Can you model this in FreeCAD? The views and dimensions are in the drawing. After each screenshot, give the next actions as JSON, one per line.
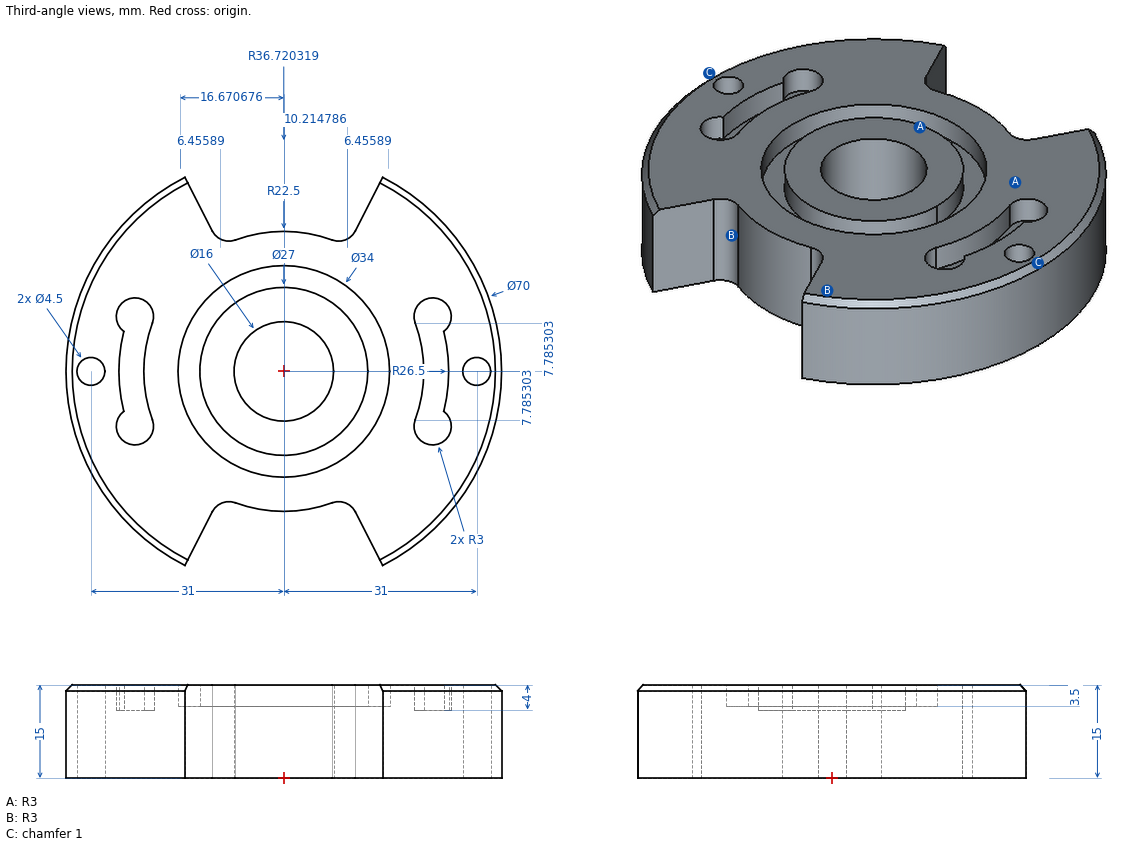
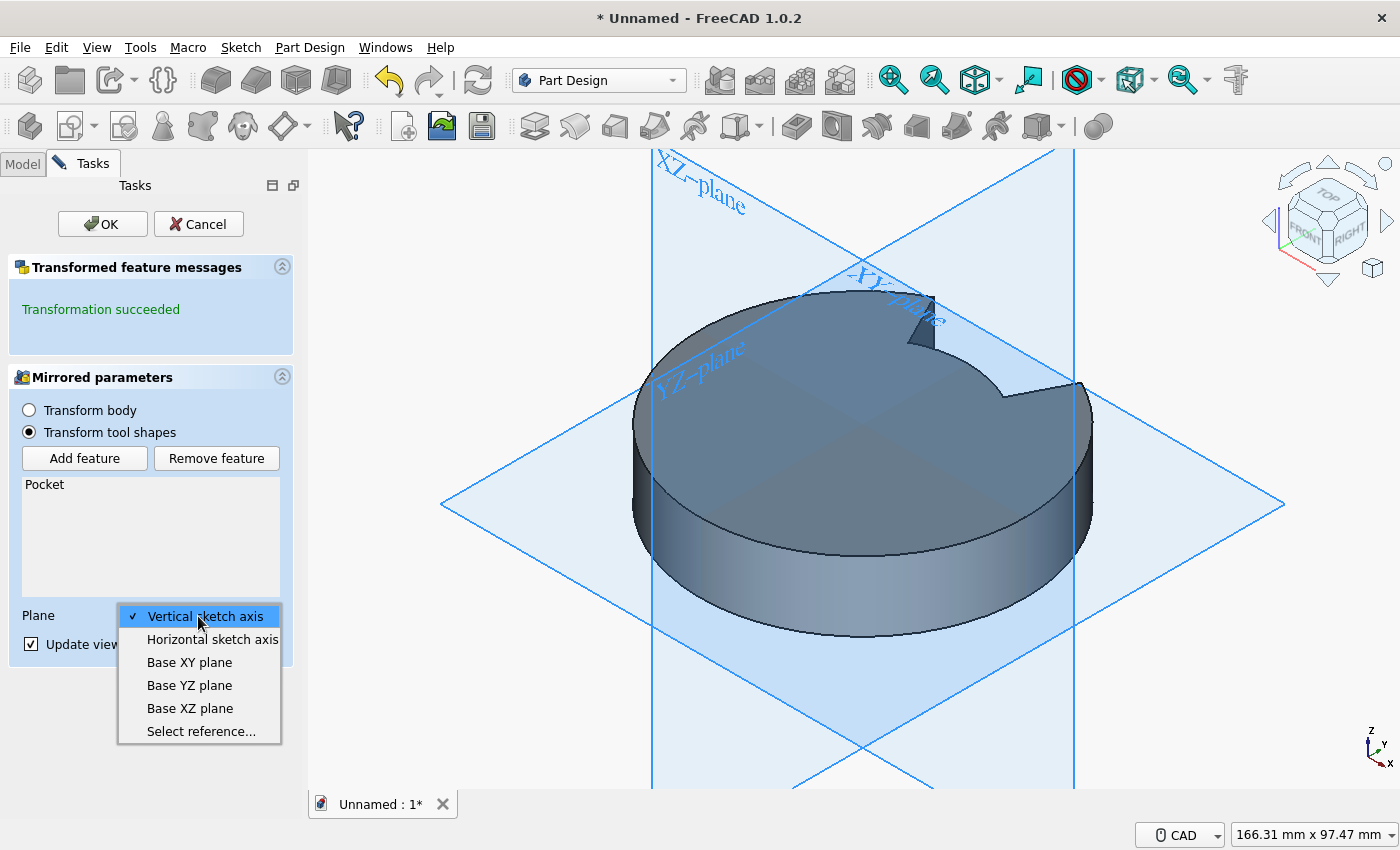
{"action": "left_click", "coordinate": [198, 708]}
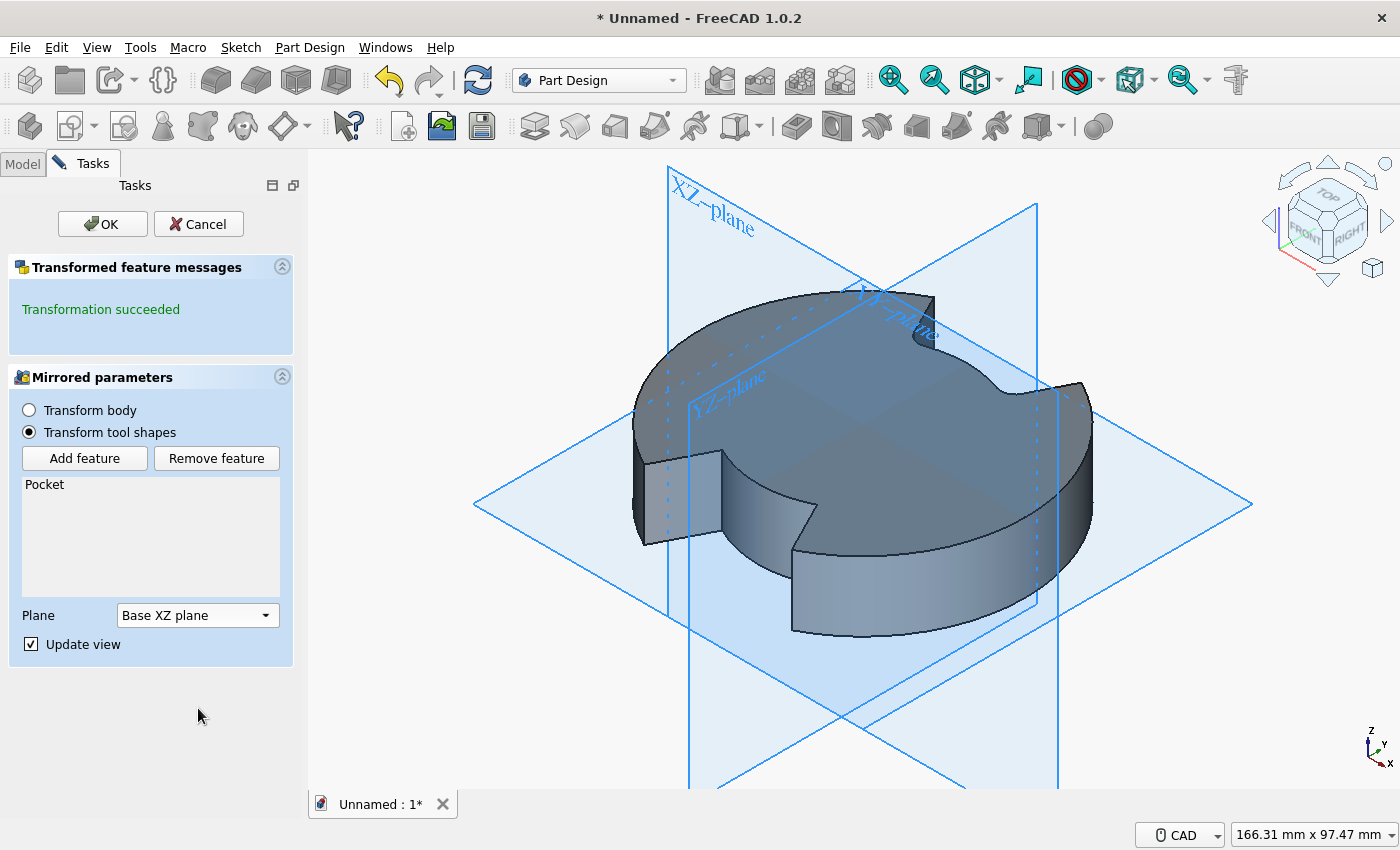
{"action": "left_click", "coordinate": [103, 224]}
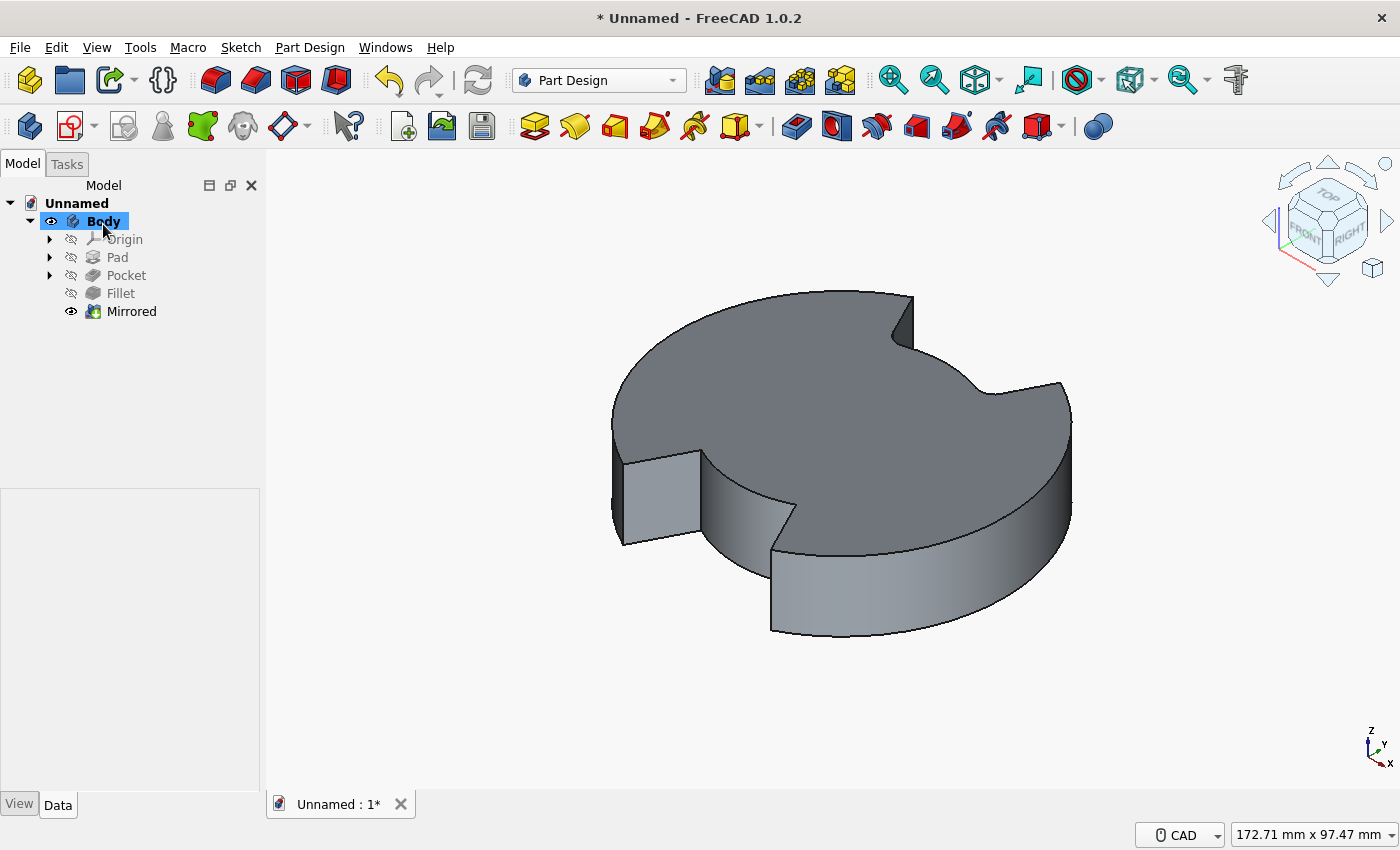
{"action": "key", "text": "2"}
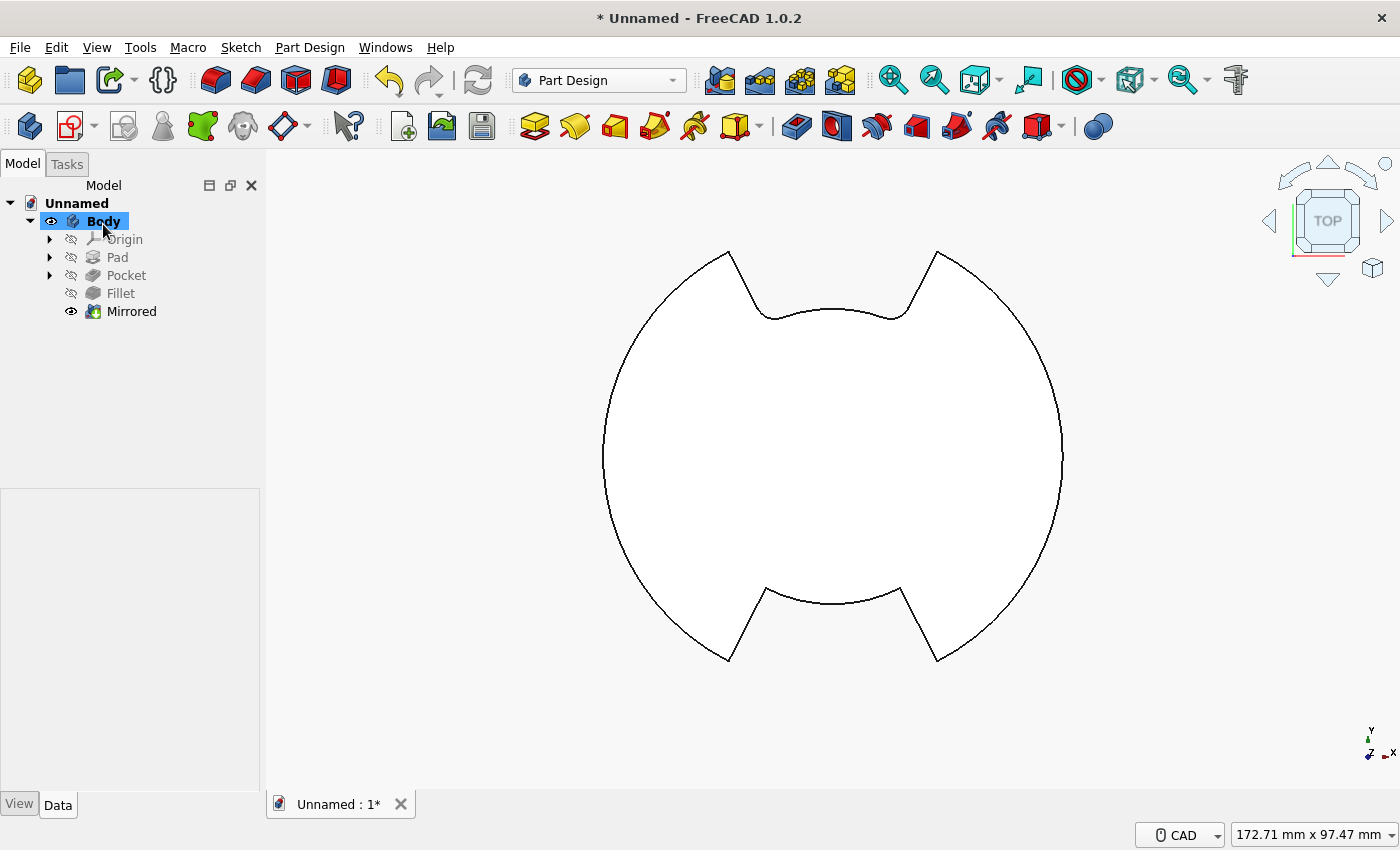
{"action": "key", "text": "0"}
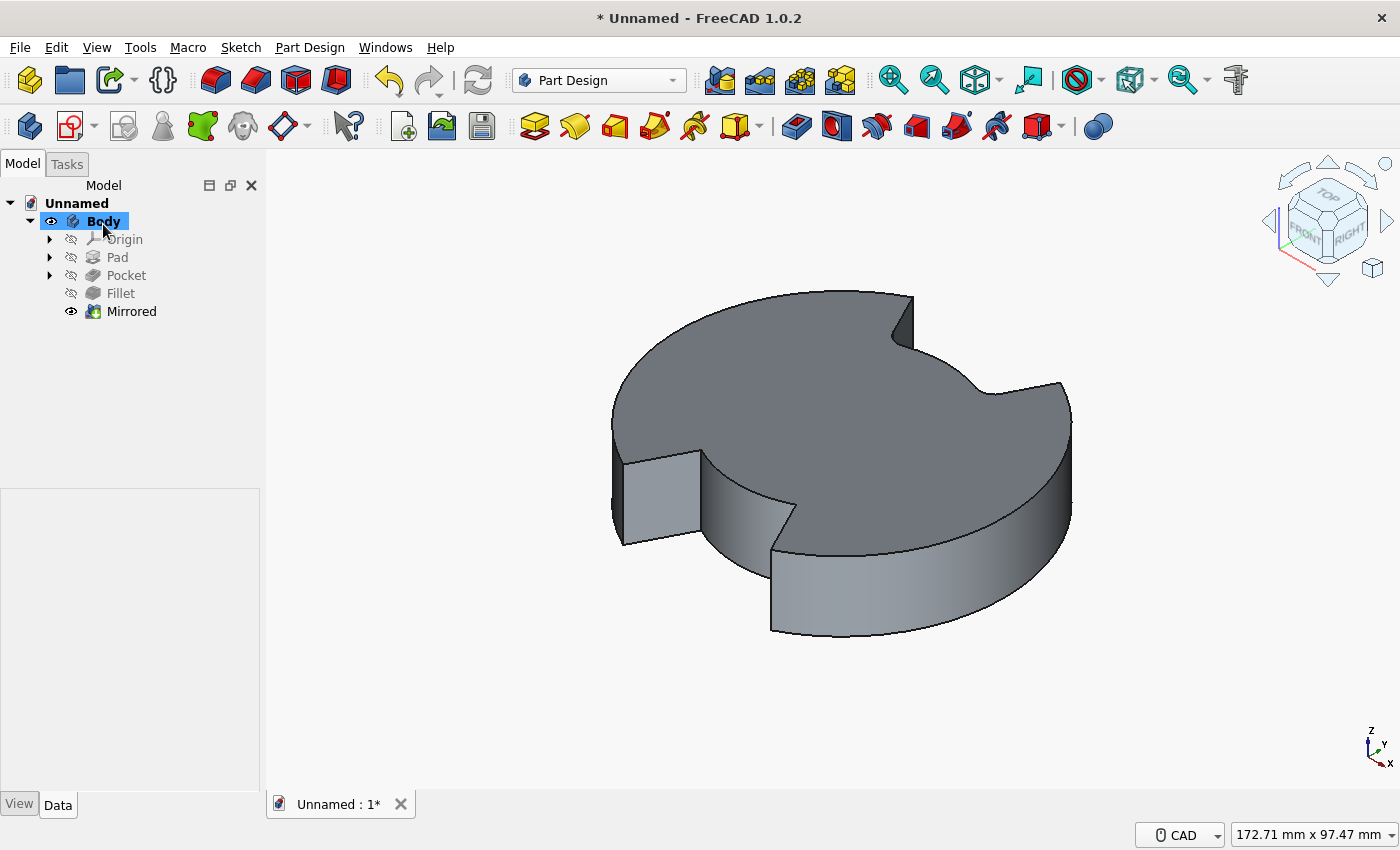
{"action": "key", "text": "1"}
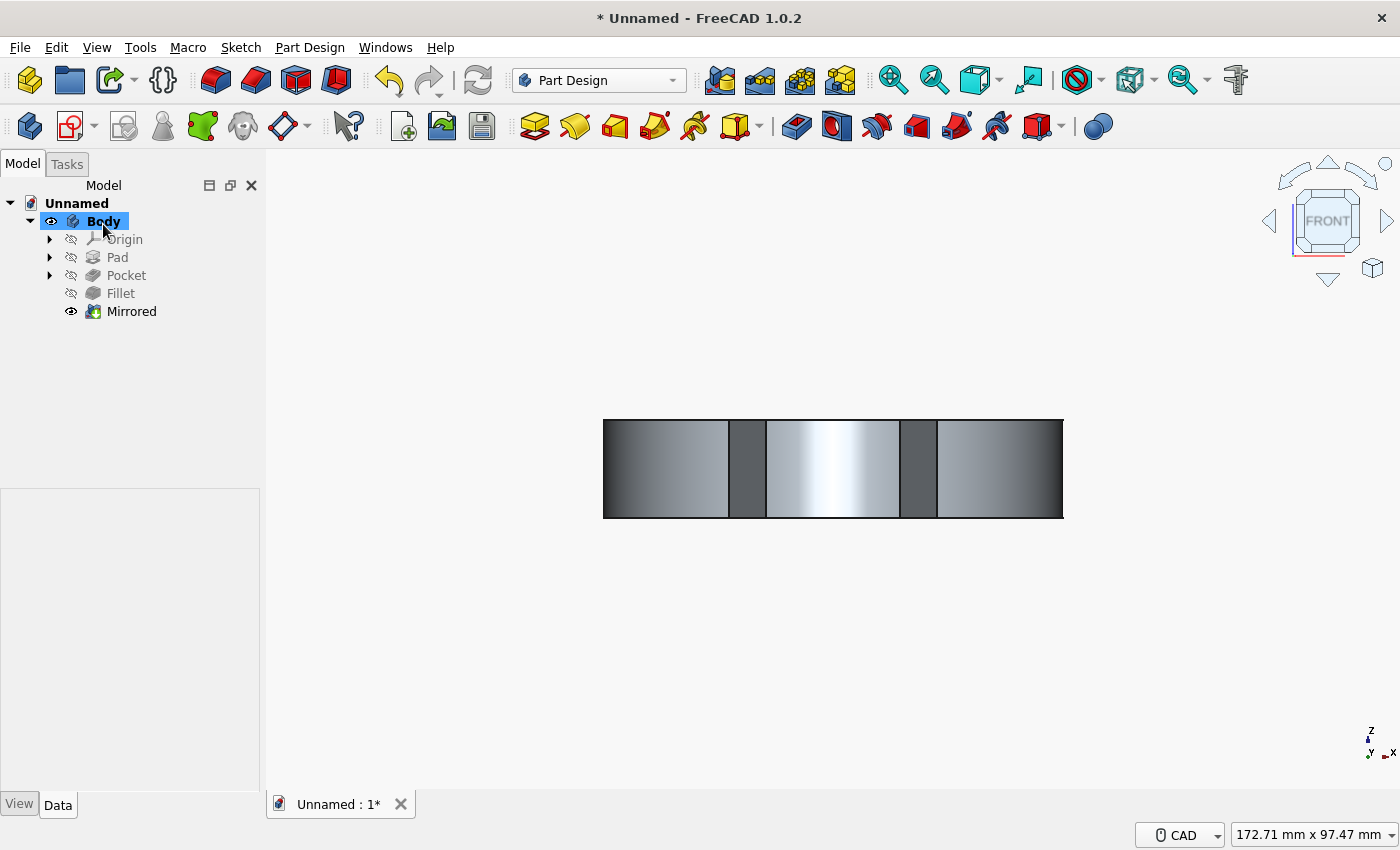
{"action": "left_click", "coordinate": [894, 80]}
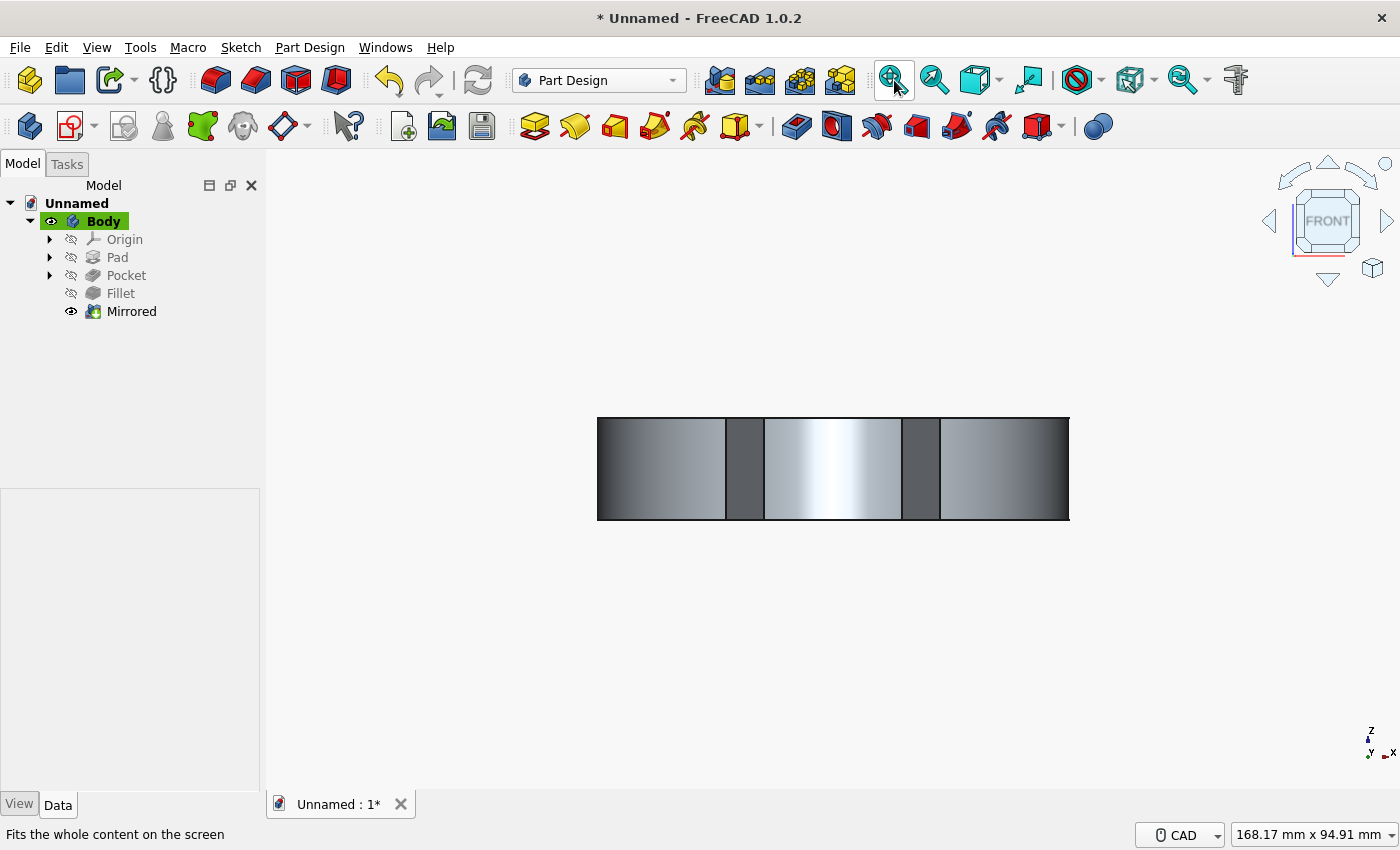
{"action": "key", "text": "3"}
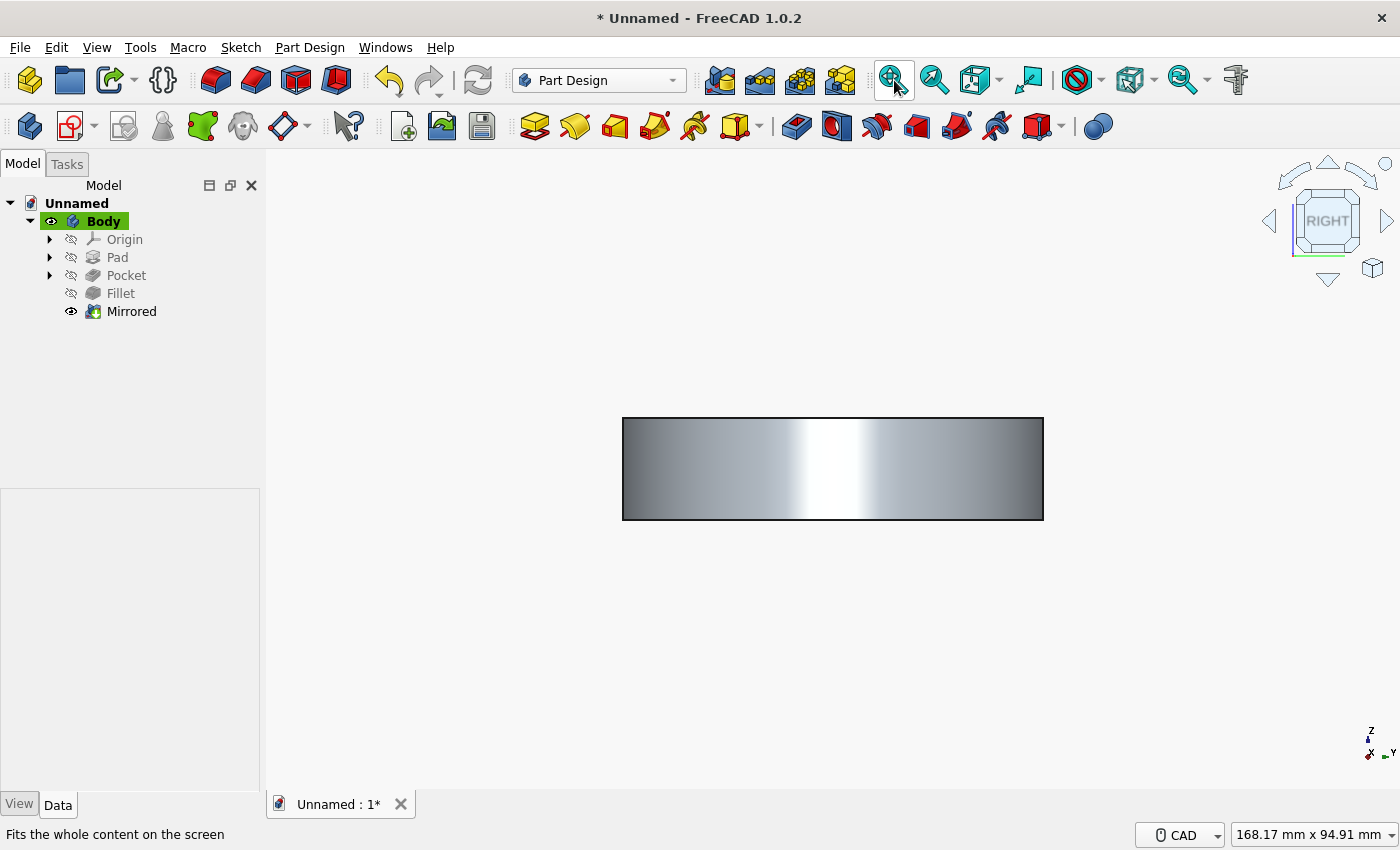
{"action": "left_click", "coordinate": [894, 80]}